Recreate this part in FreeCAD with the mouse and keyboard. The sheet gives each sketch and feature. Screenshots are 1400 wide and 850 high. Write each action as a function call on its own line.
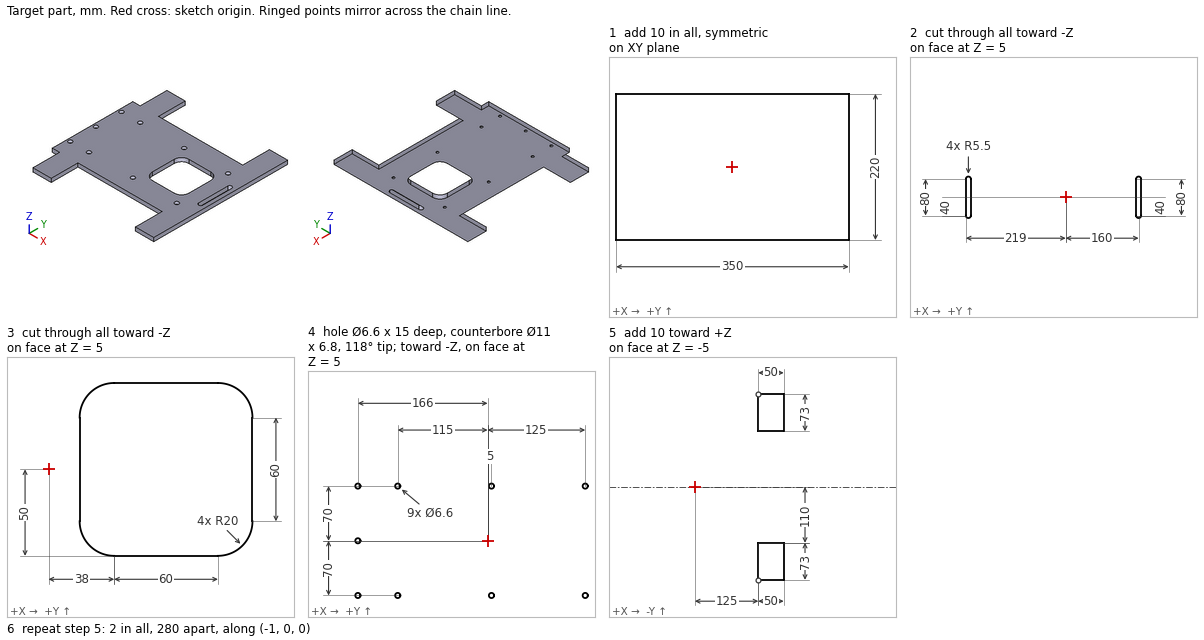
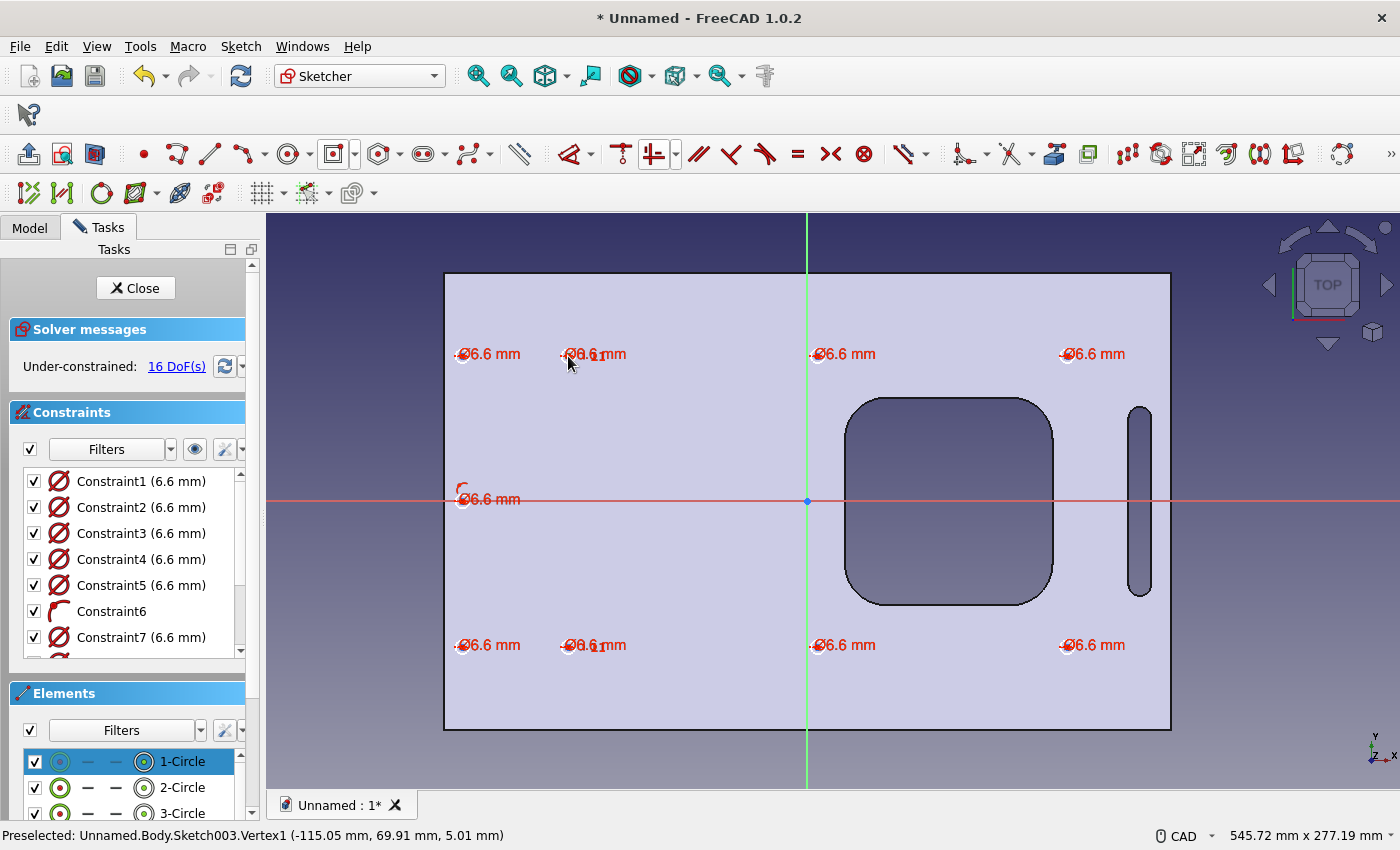
click(462, 356)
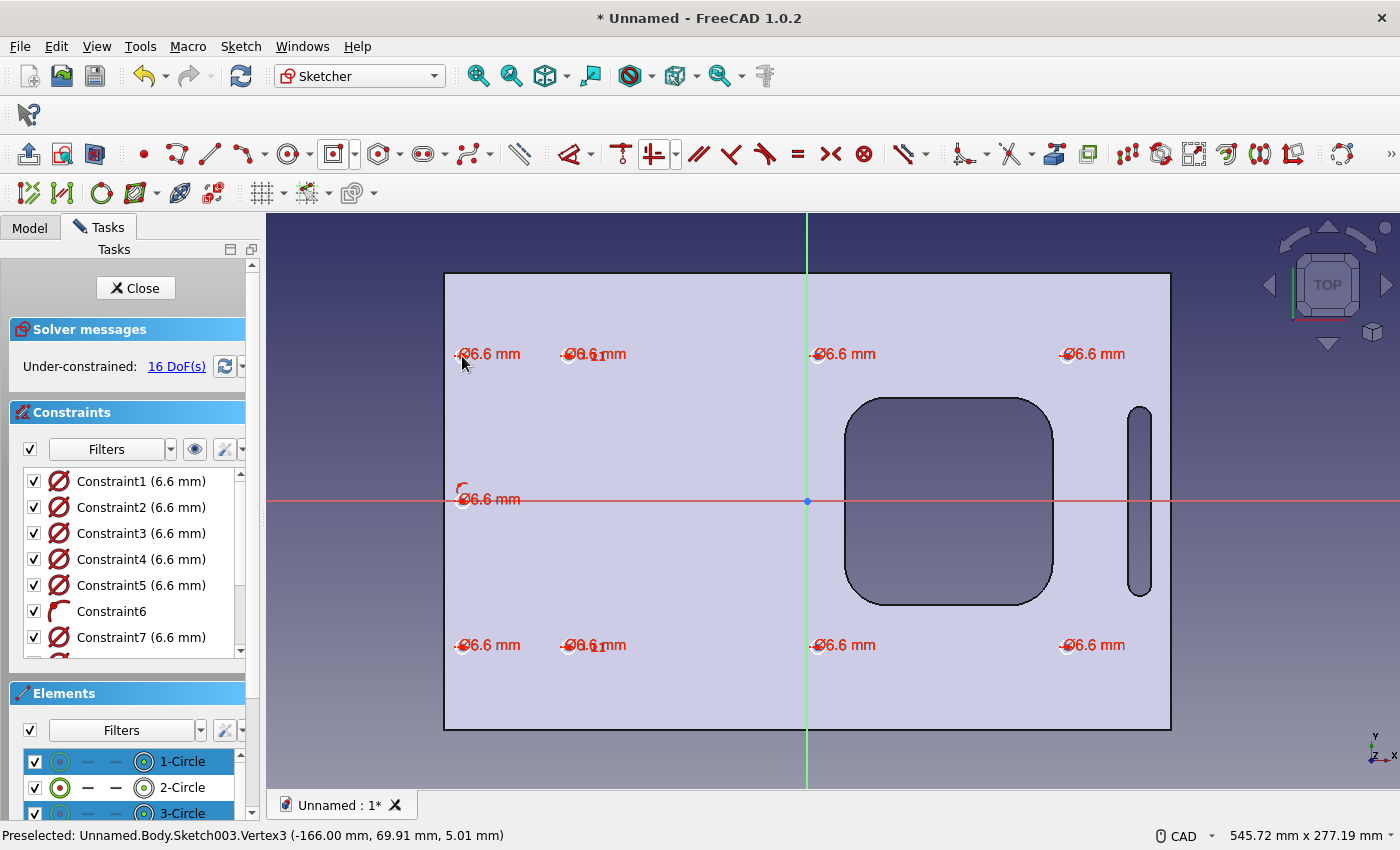
key(h)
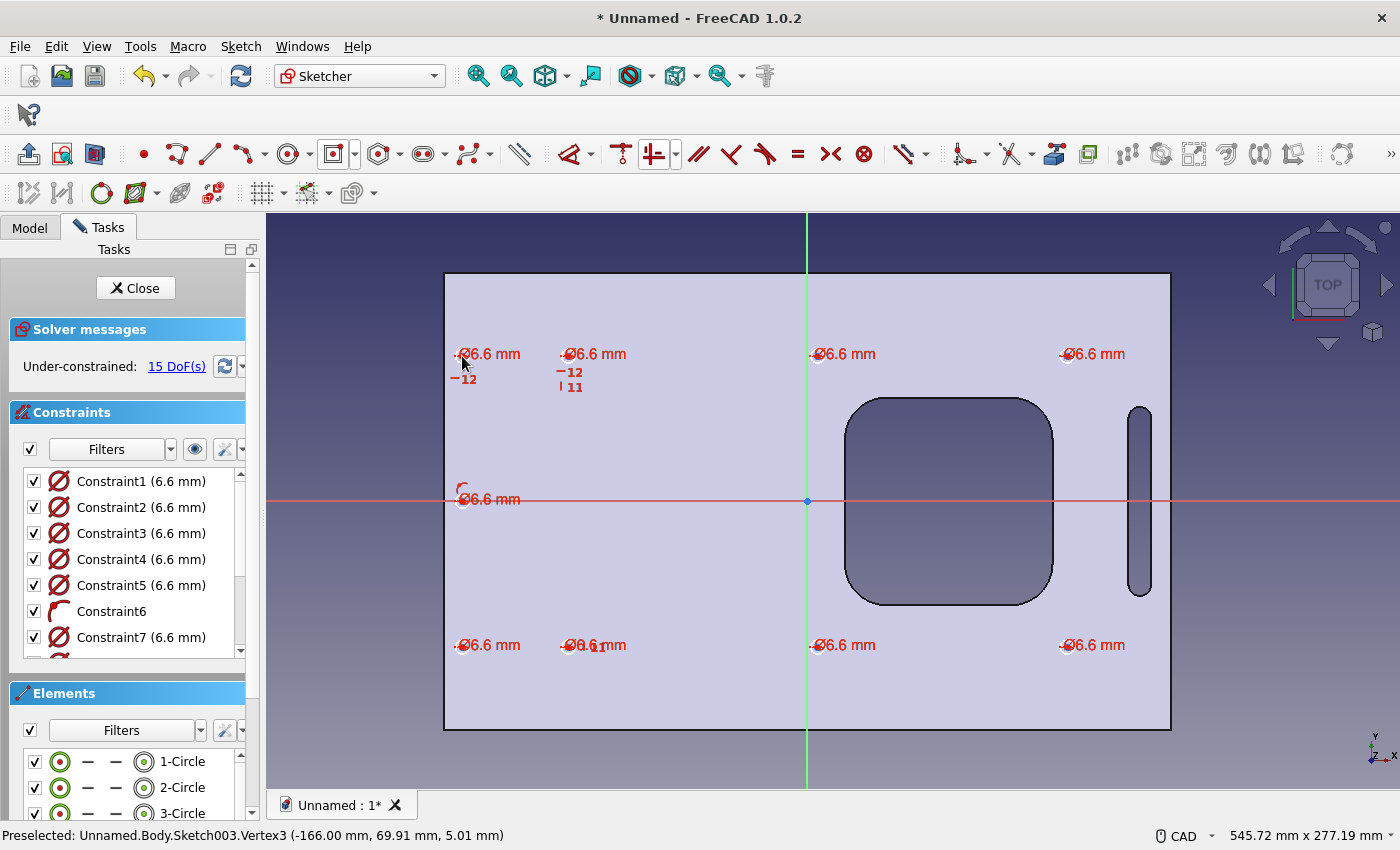
click(462, 356)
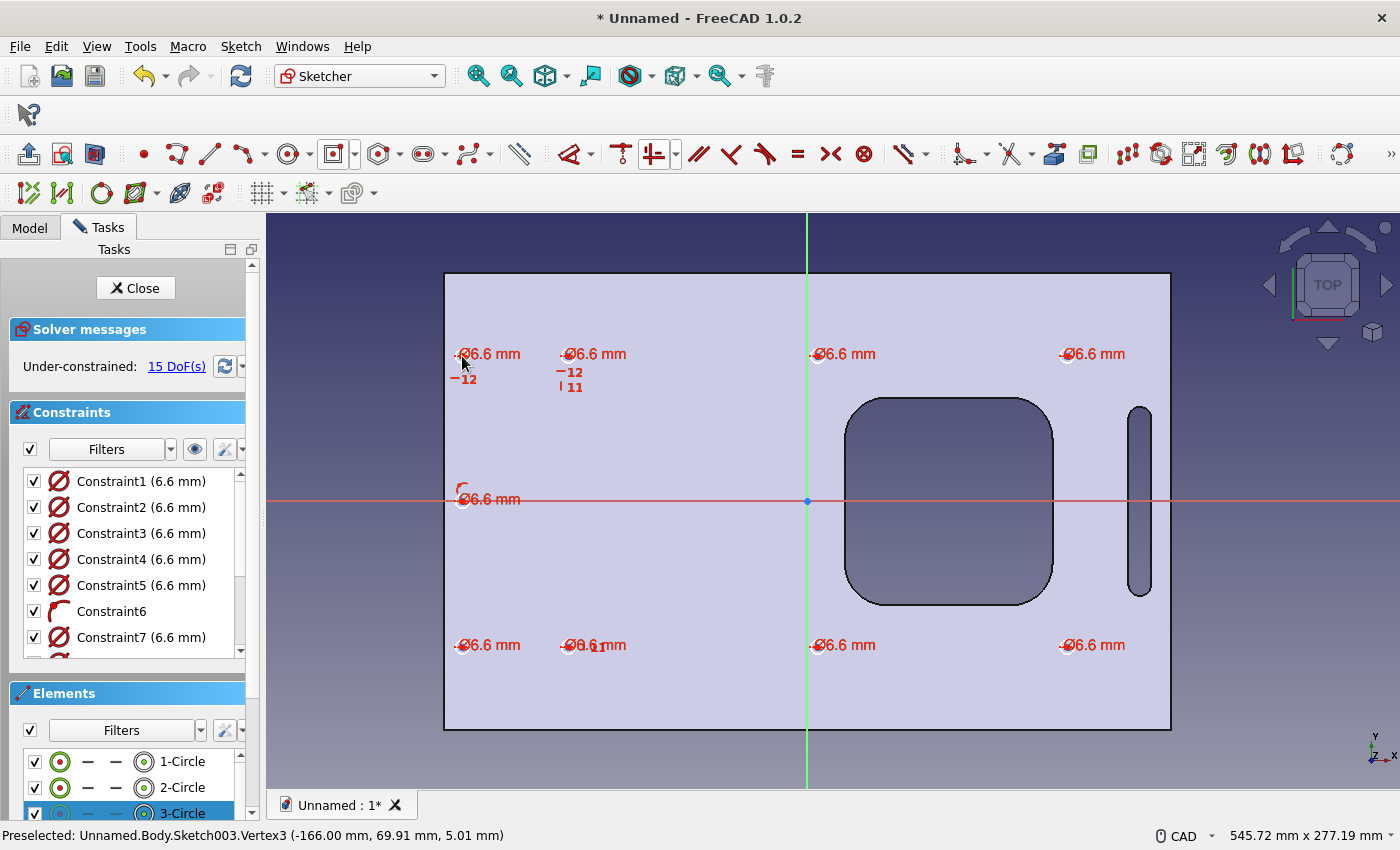
click(462, 647)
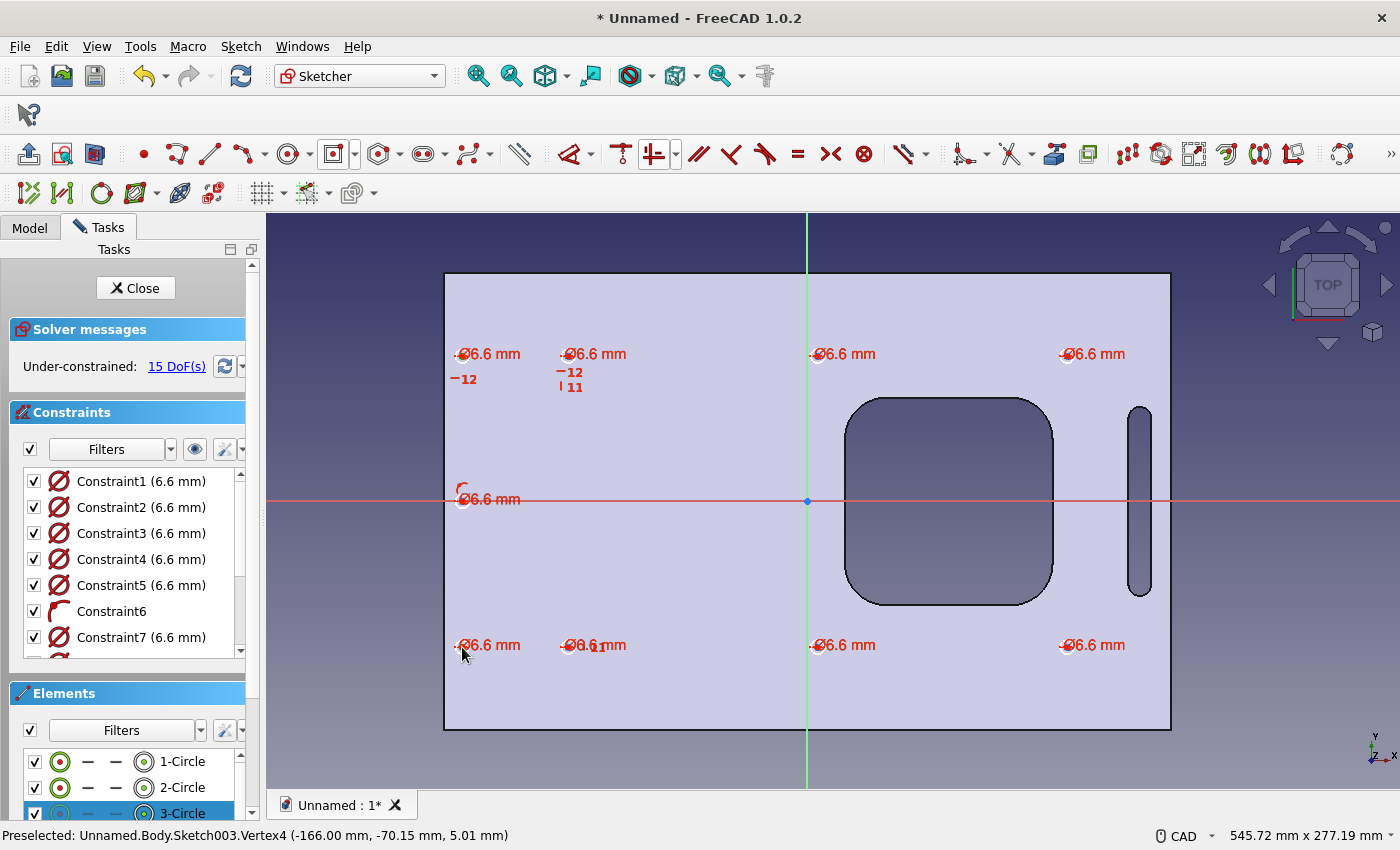
key(v)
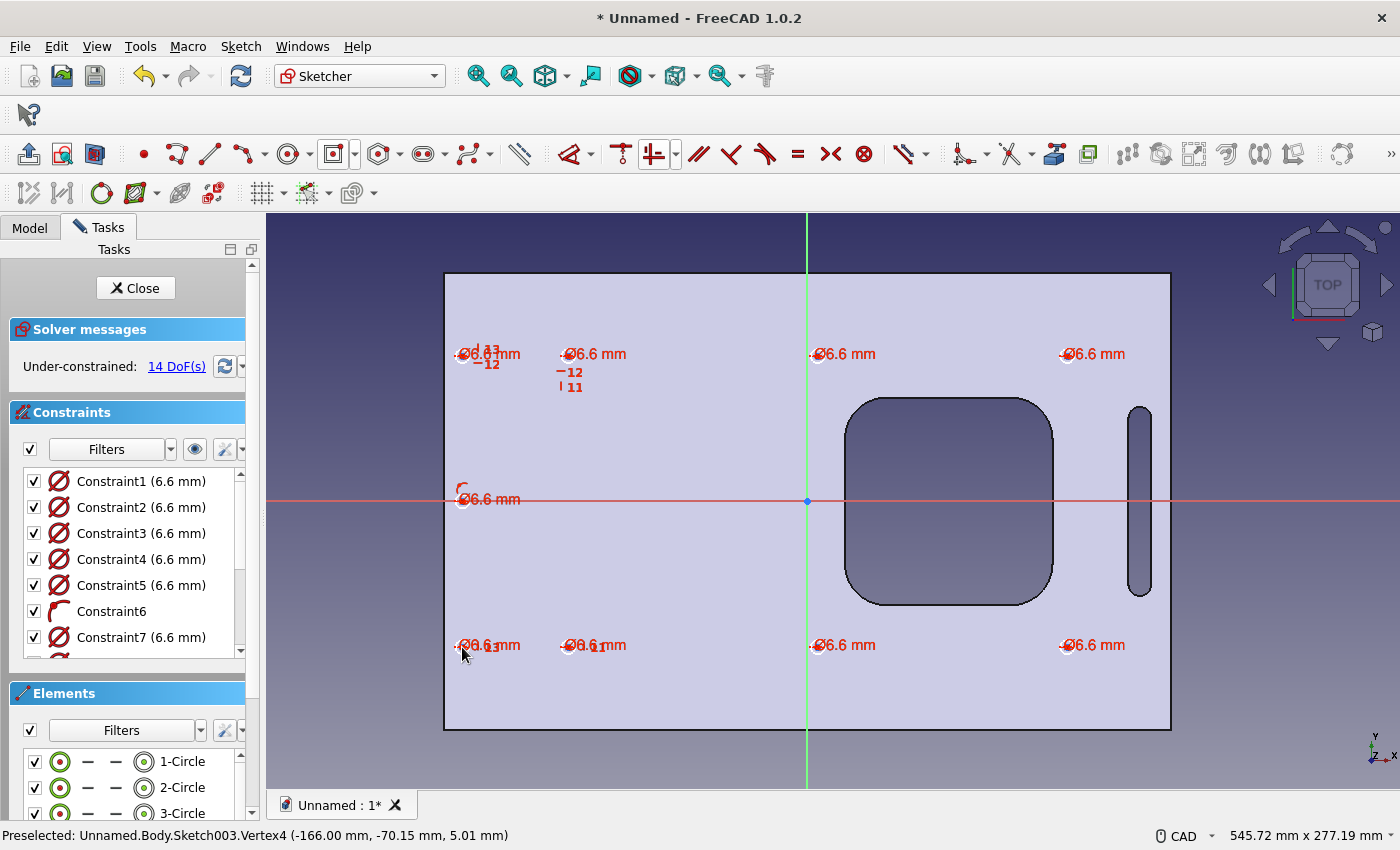
click(568, 647)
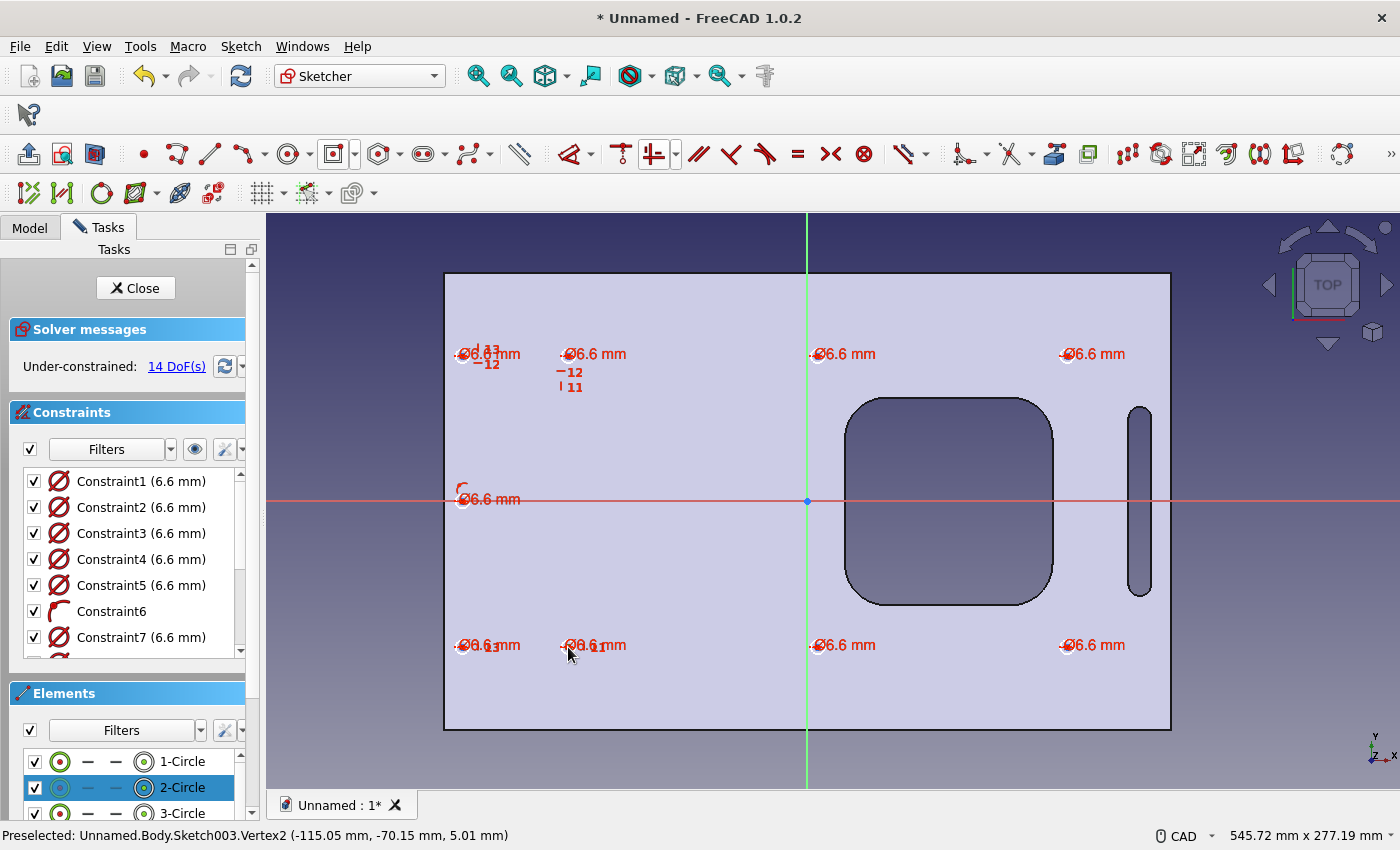
click(462, 647)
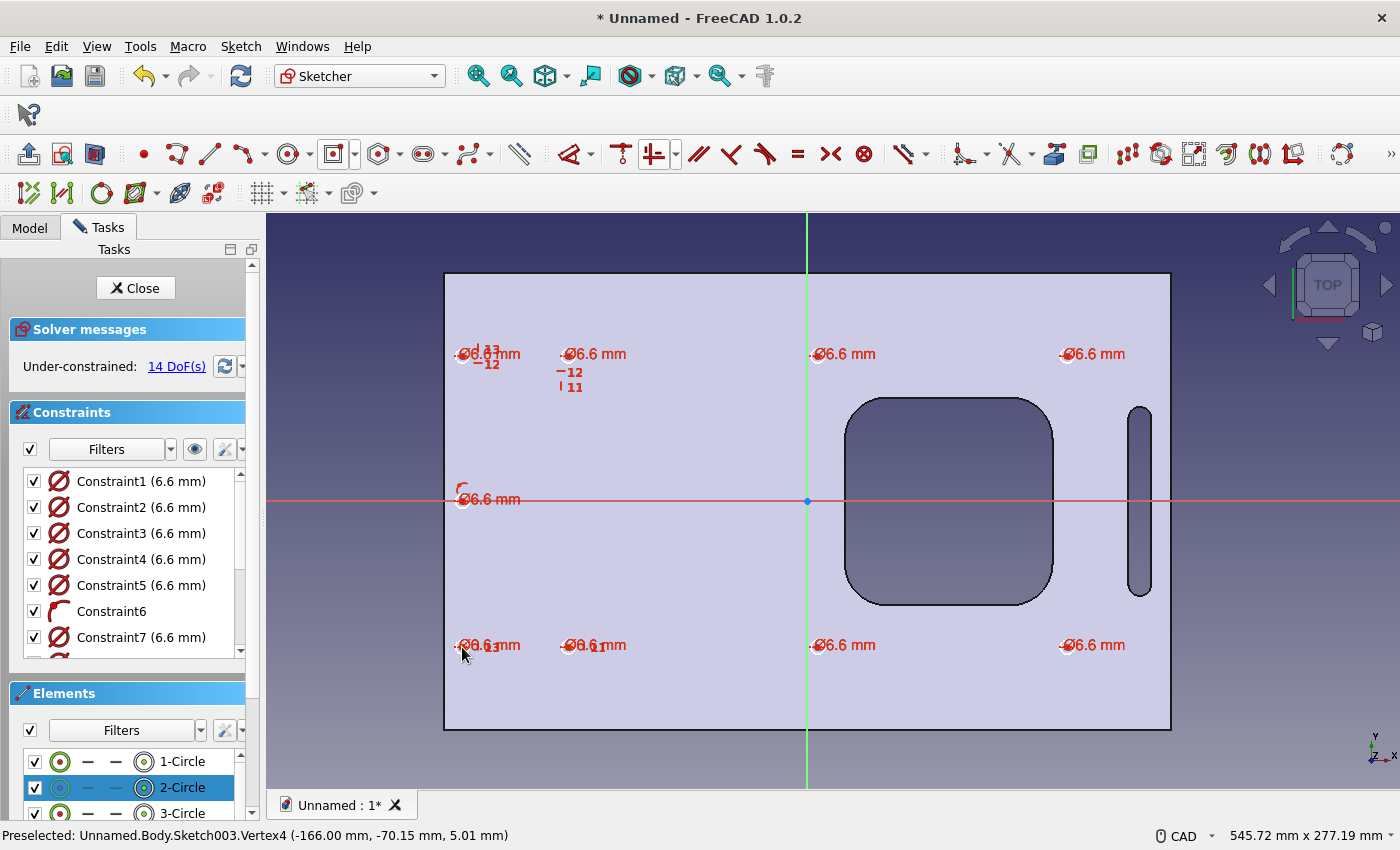
key(h)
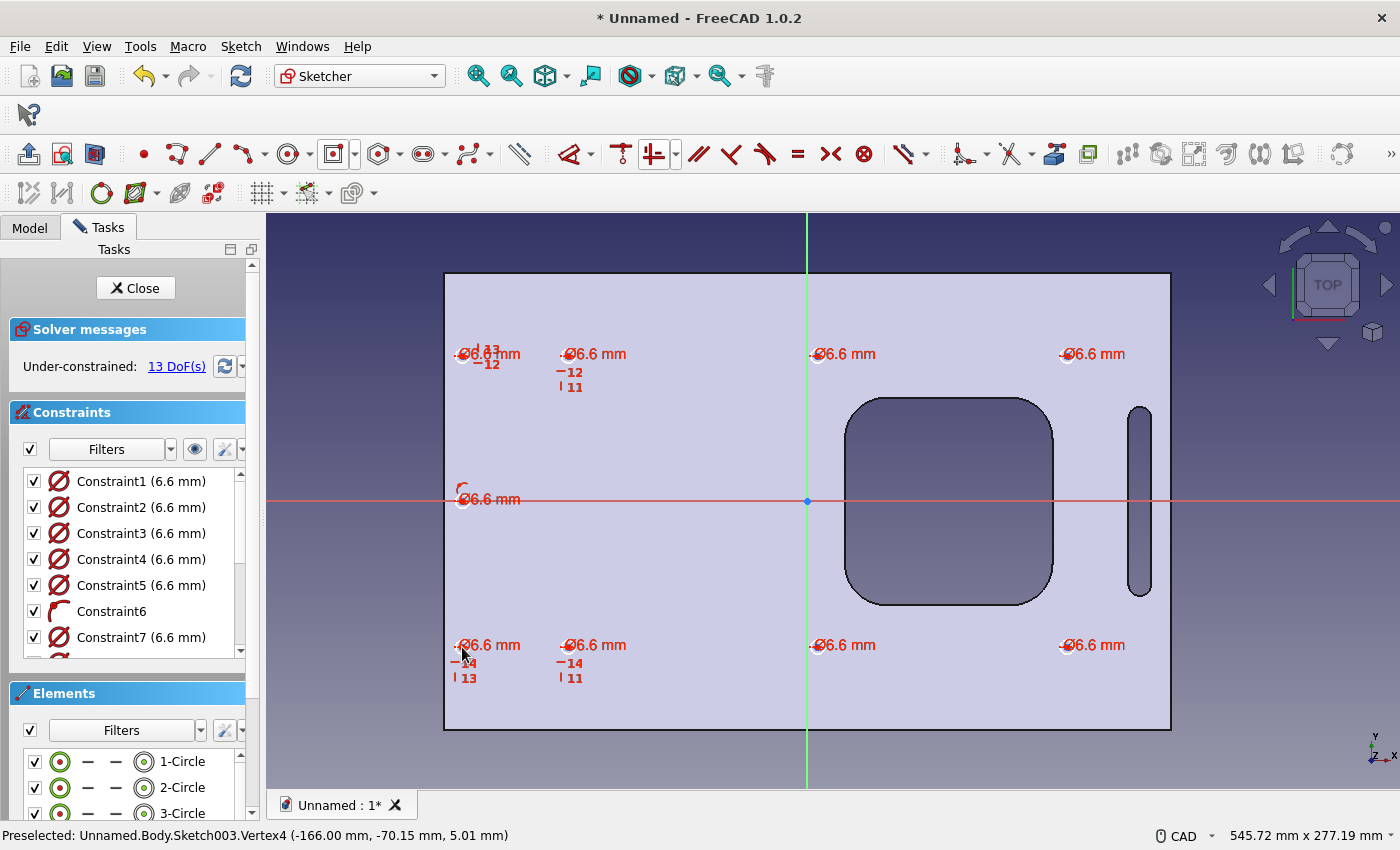
click(462, 356)